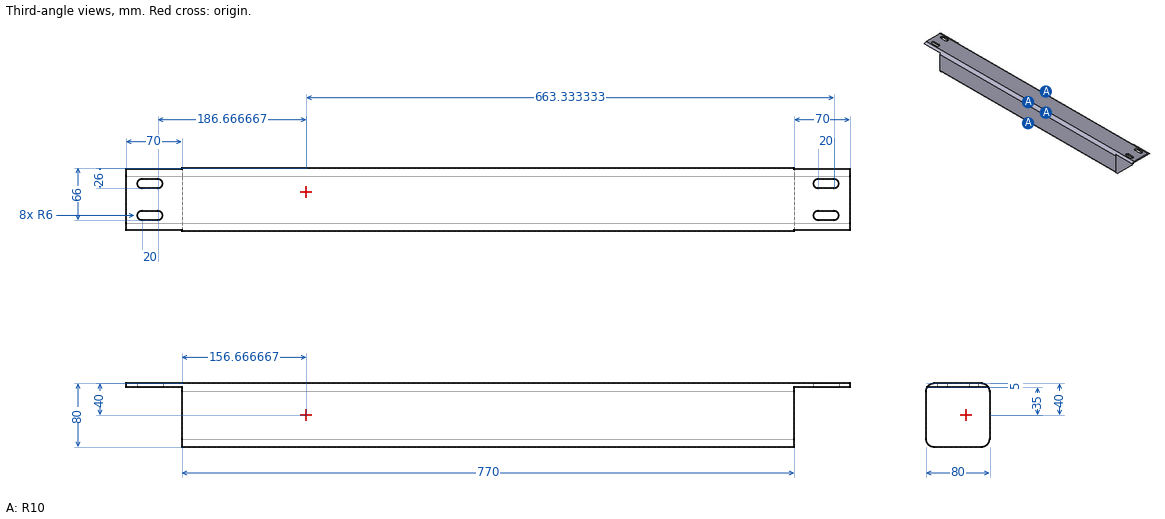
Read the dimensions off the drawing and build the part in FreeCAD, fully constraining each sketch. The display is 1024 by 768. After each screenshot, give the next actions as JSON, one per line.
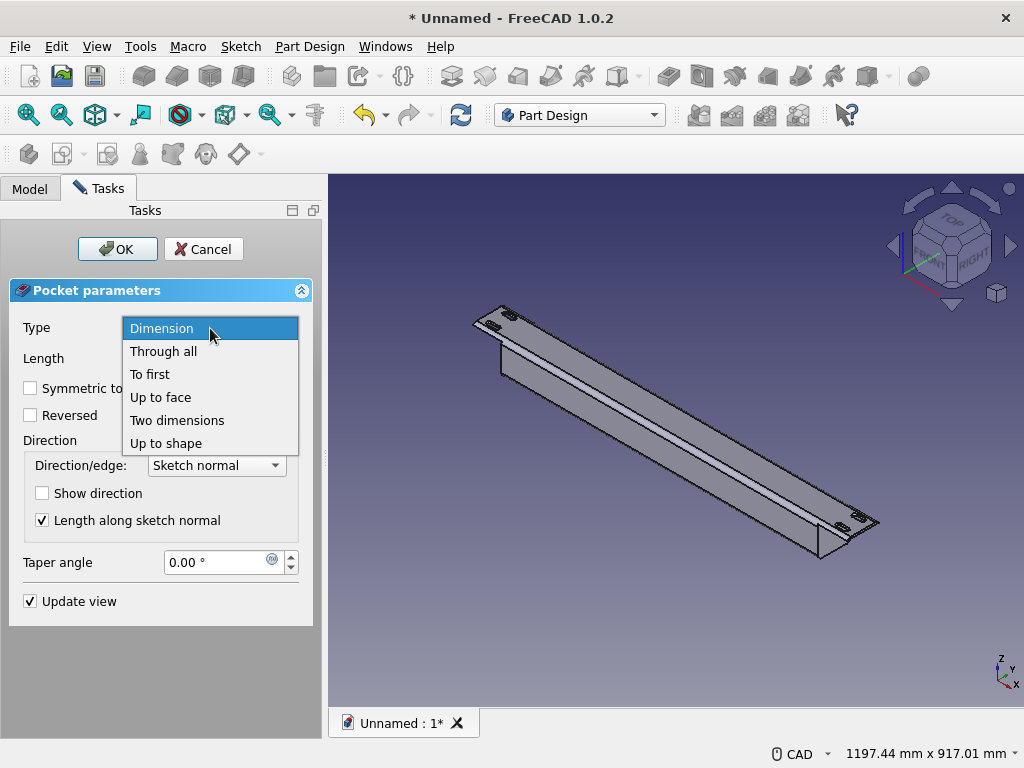
{"action": "left_click", "coordinate": [208, 352]}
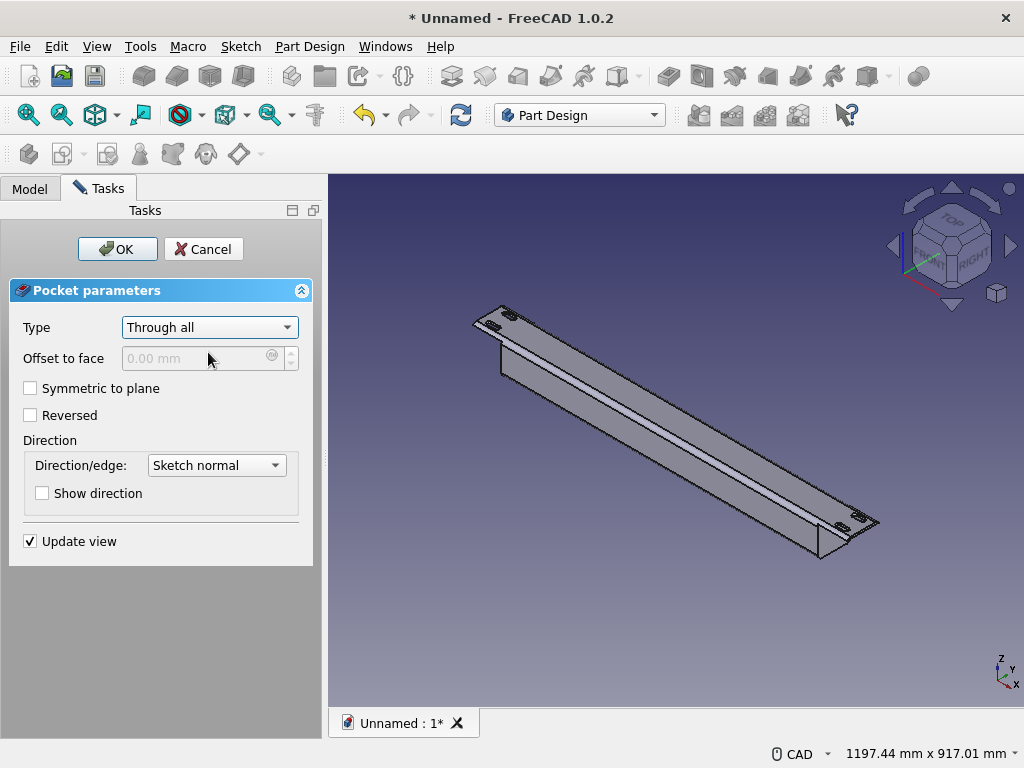
{"action": "left_click", "coordinate": [118, 249]}